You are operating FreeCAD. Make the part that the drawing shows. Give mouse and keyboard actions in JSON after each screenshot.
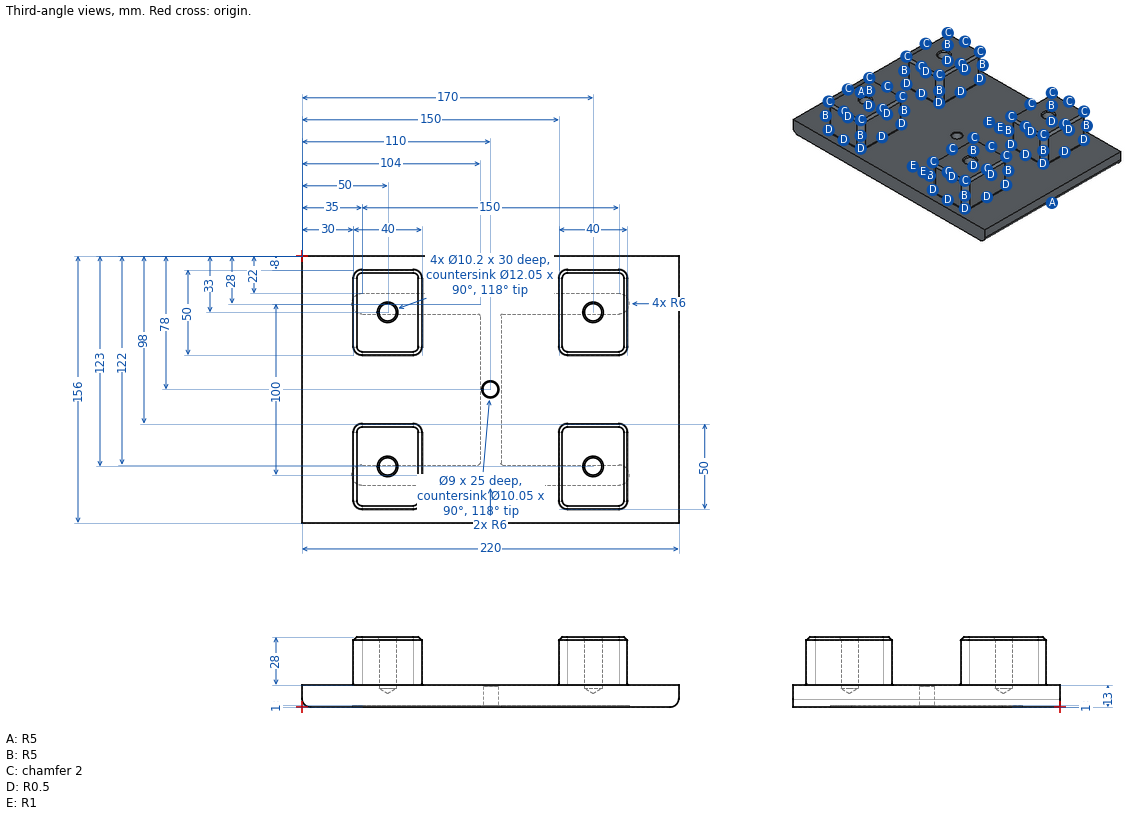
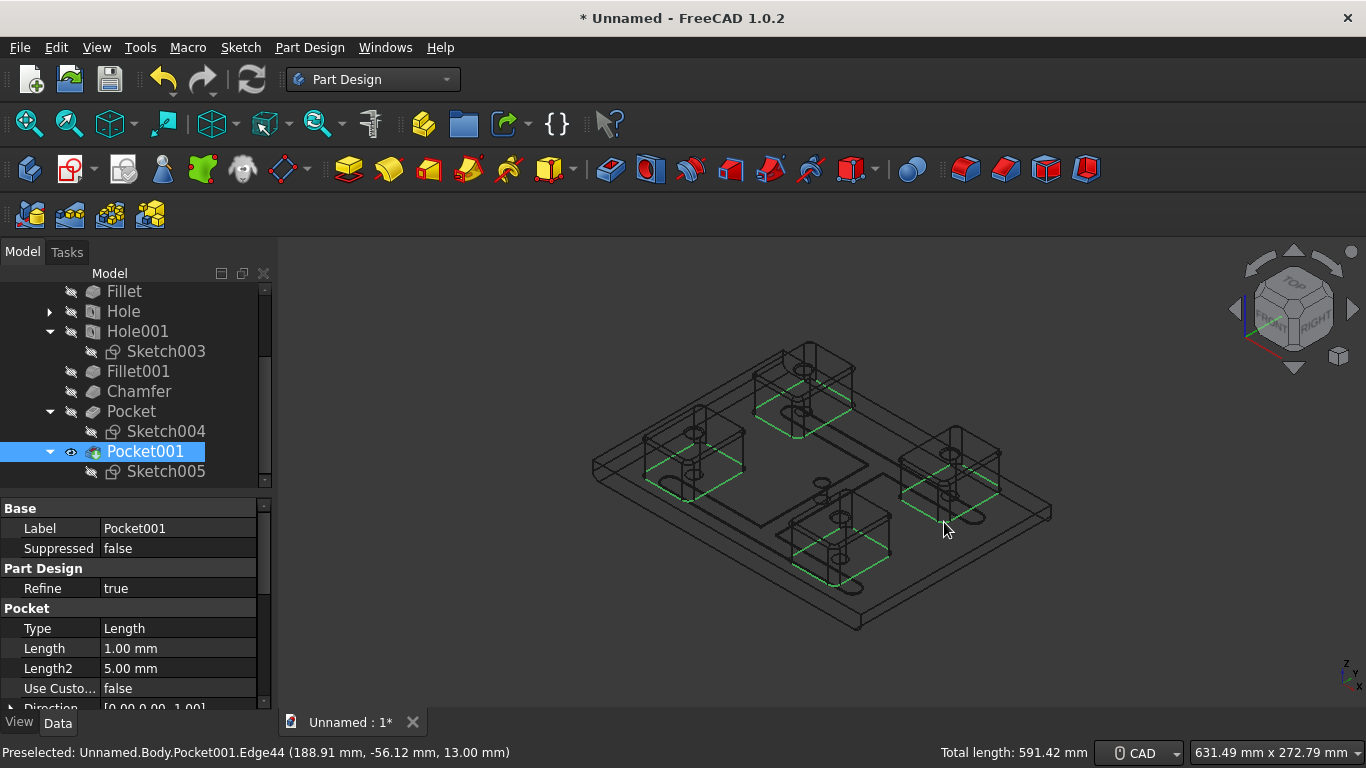
{"action": "scroll", "coordinate": [745, 467], "scroll_direction": "up", "scroll_amount": 6}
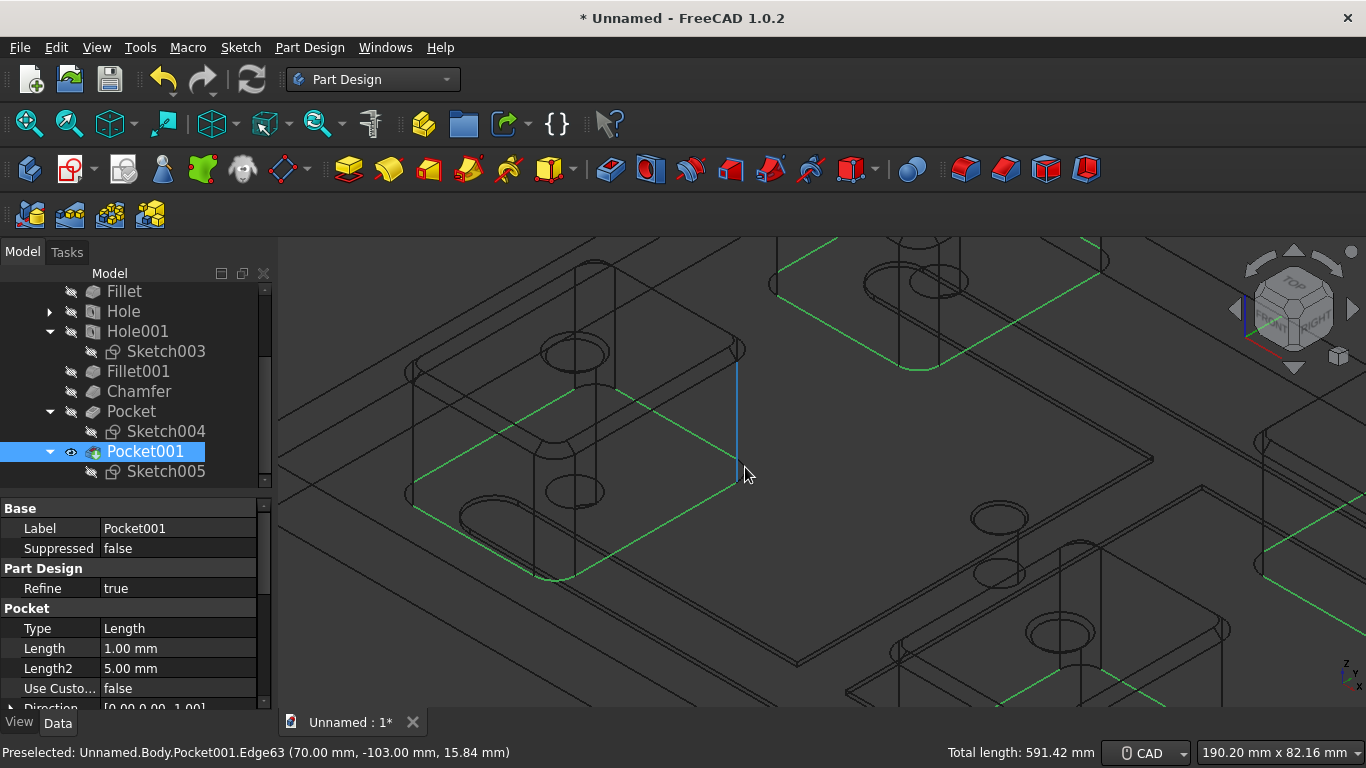
{"action": "left_click", "coordinate": [745, 470], "text": "ctrl"}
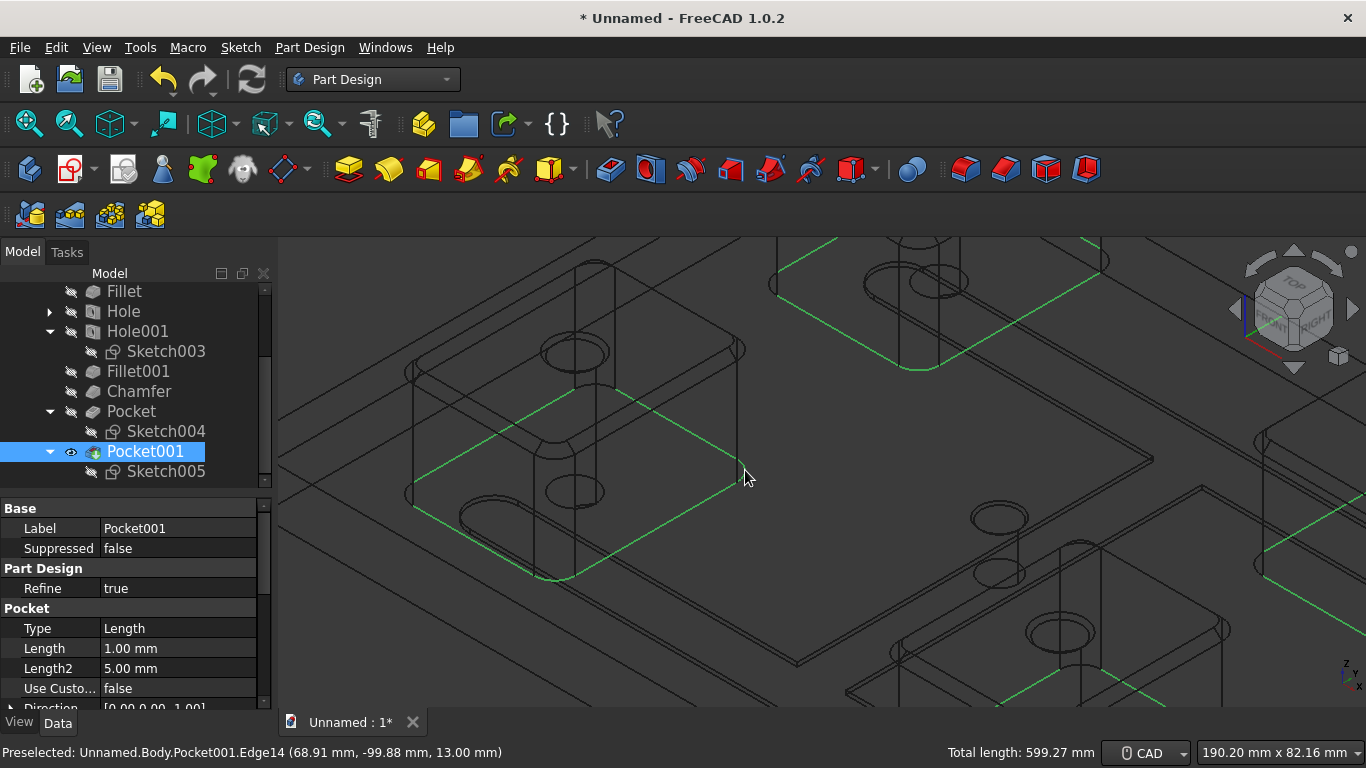
{"action": "left_click", "coordinate": [586, 384], "text": "ctrl"}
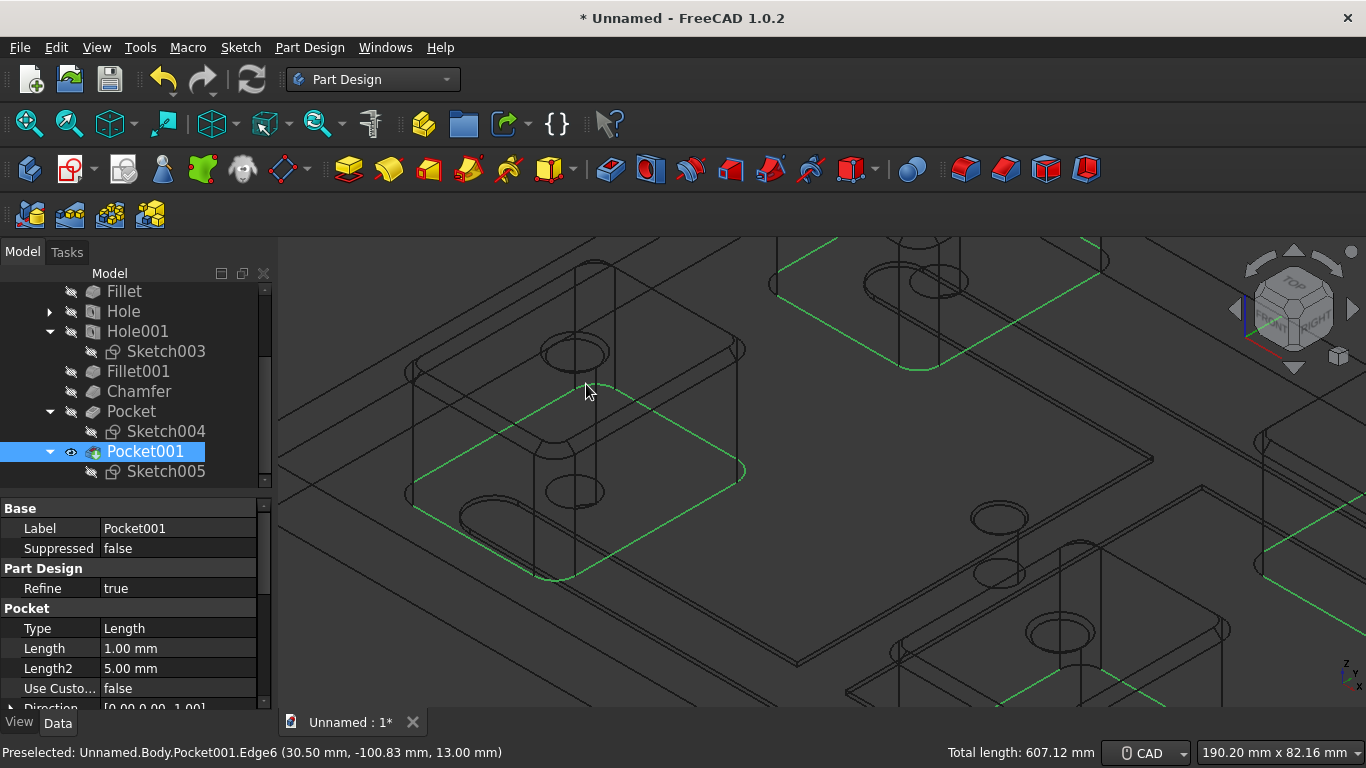
{"action": "left_click", "coordinate": [405, 493], "text": "ctrl"}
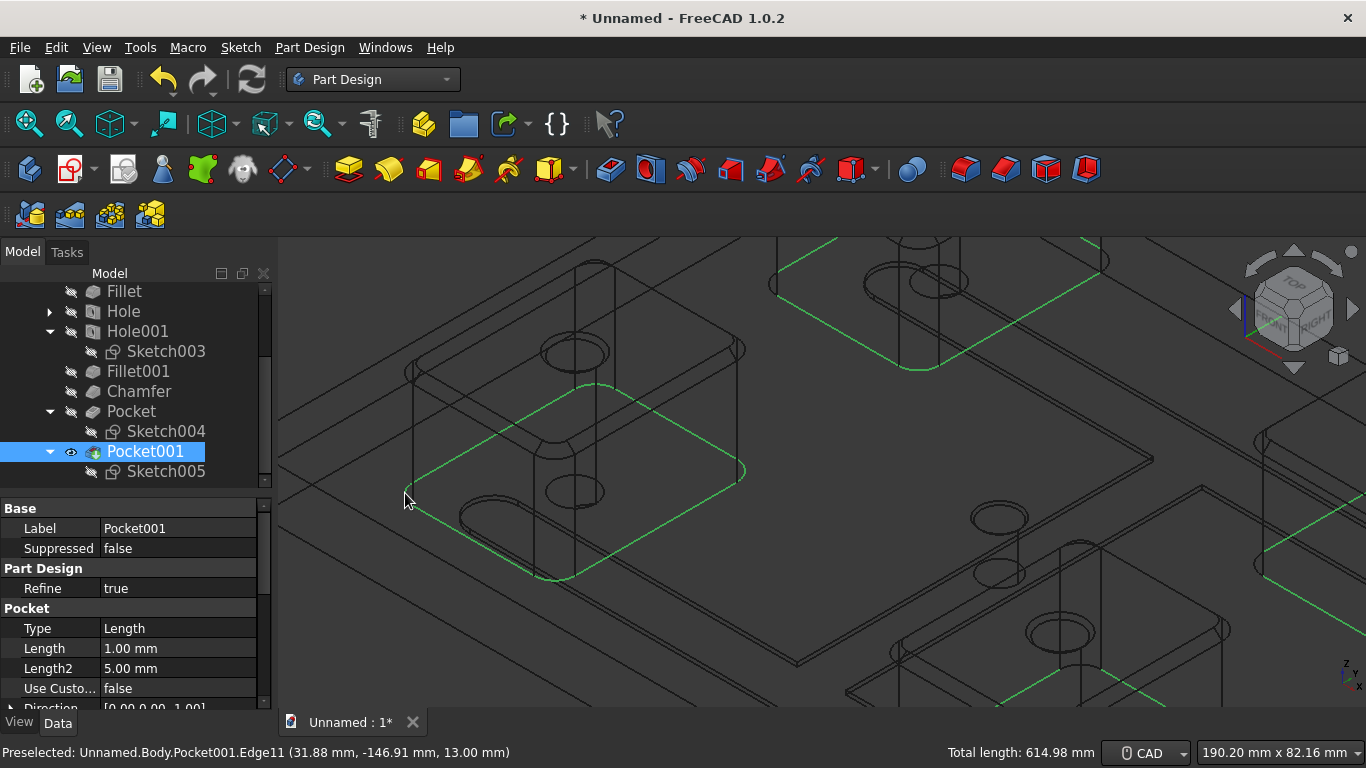
{"action": "left_click", "coordinate": [1072, 664], "text": "ctrl"}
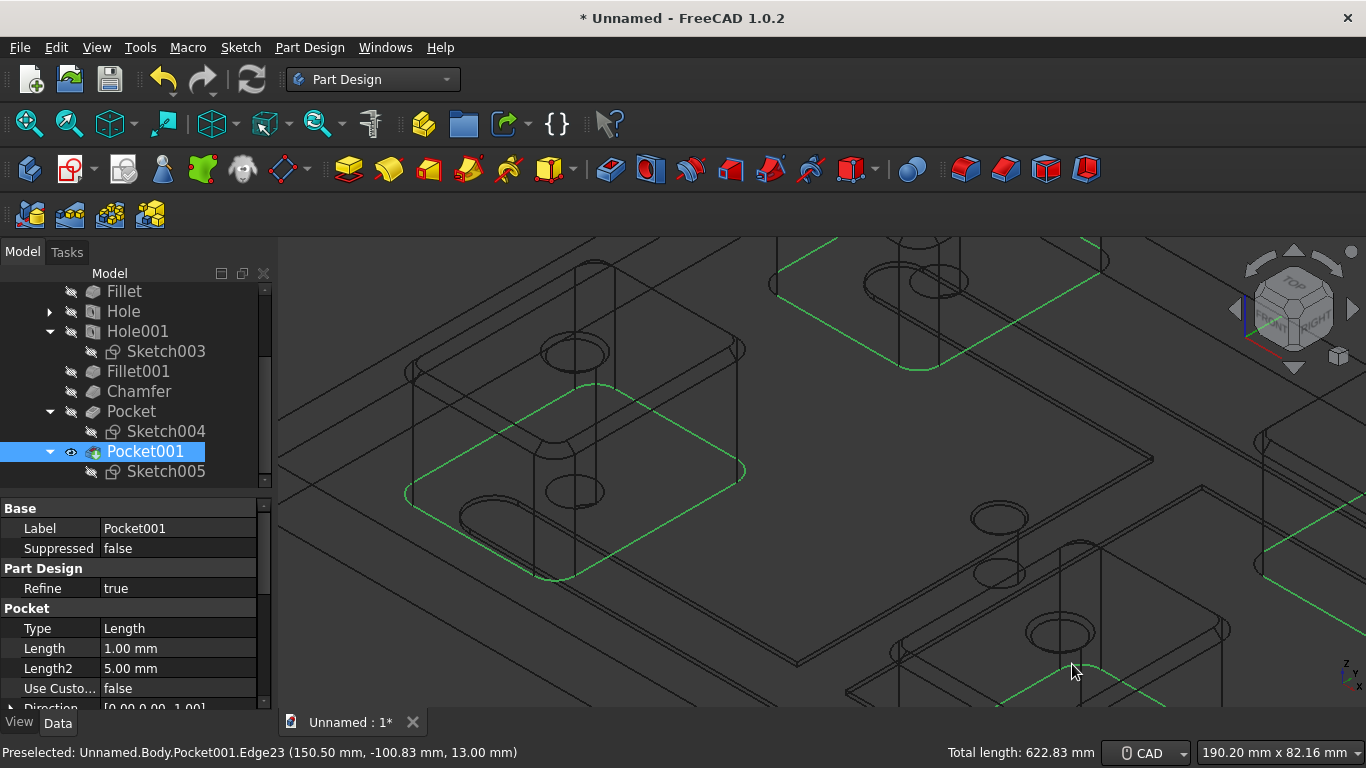
{"action": "left_click", "coordinate": [1254, 563], "text": "ctrl"}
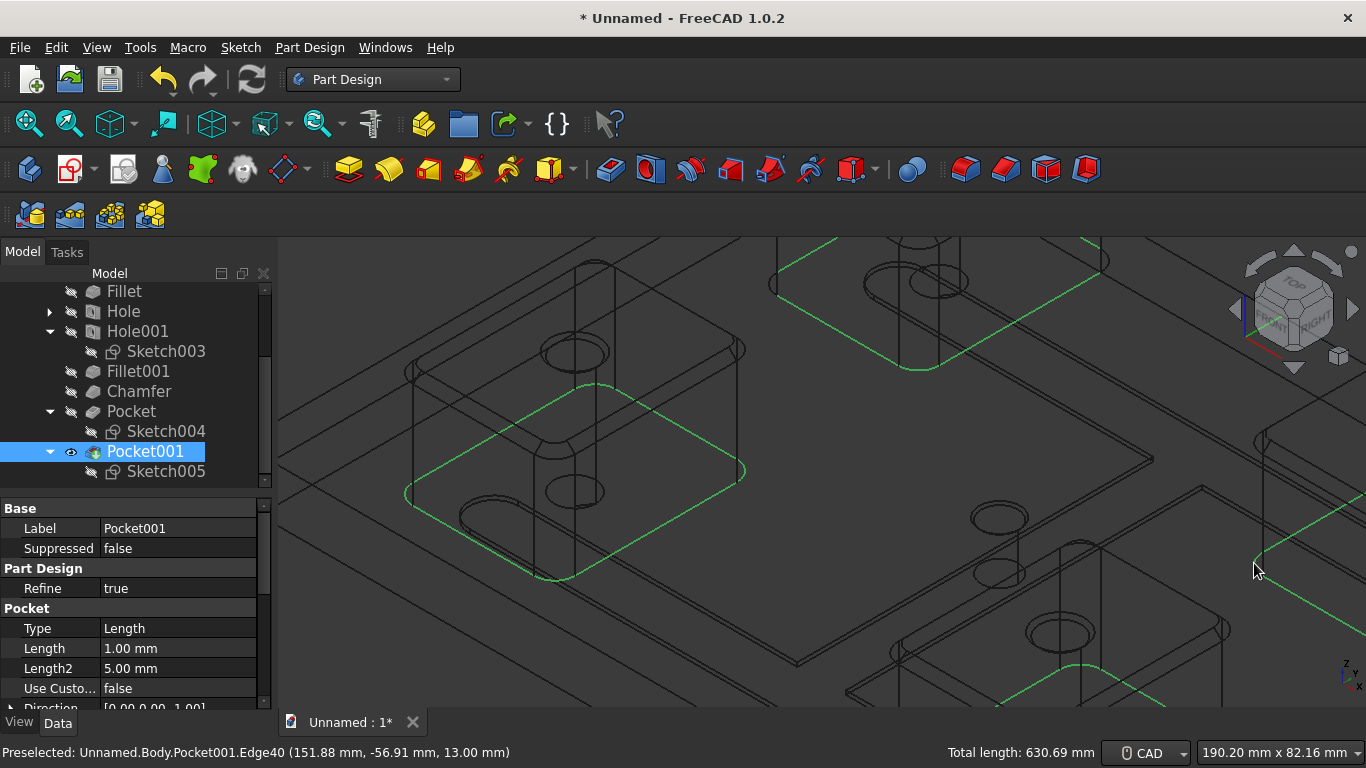
{"action": "left_click", "coordinate": [769, 283], "text": "ctrl"}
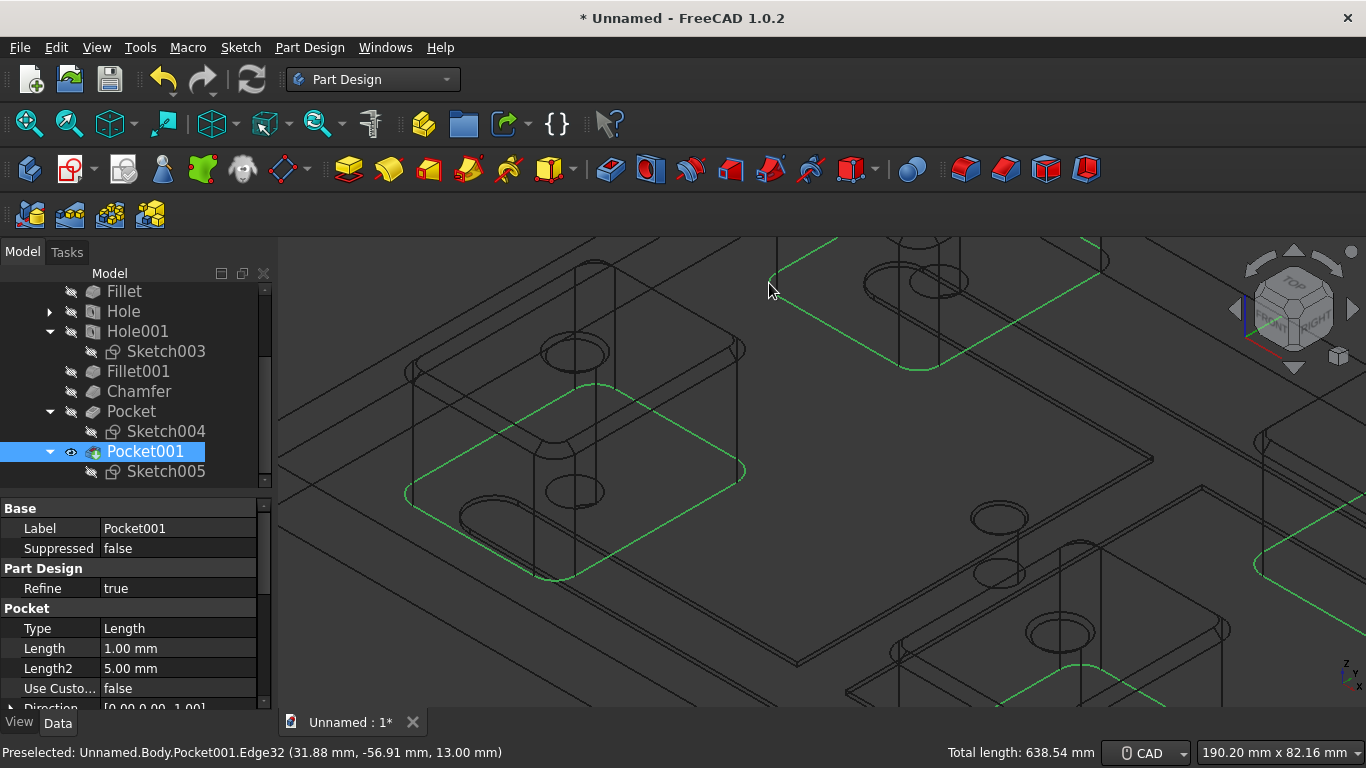
{"action": "key", "text": "v f"}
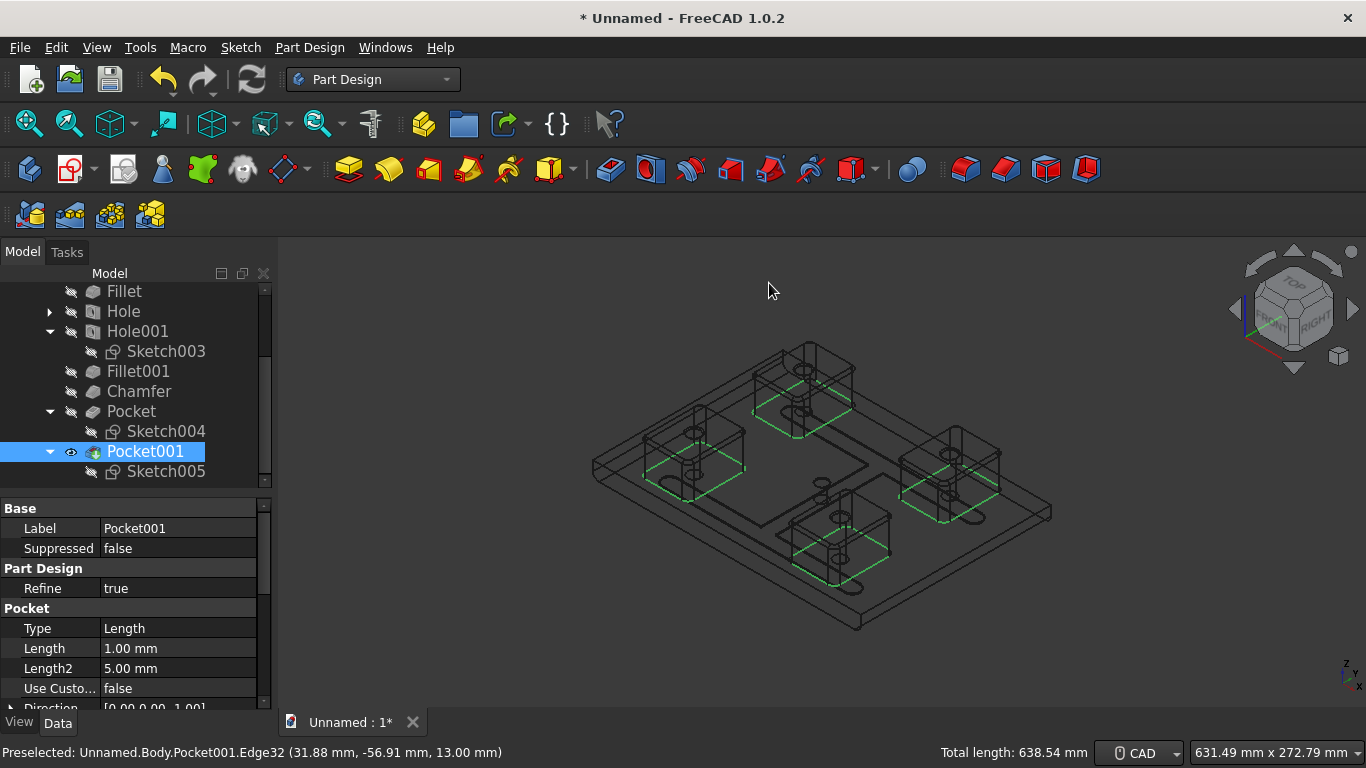
{"action": "key", "text": "2"}